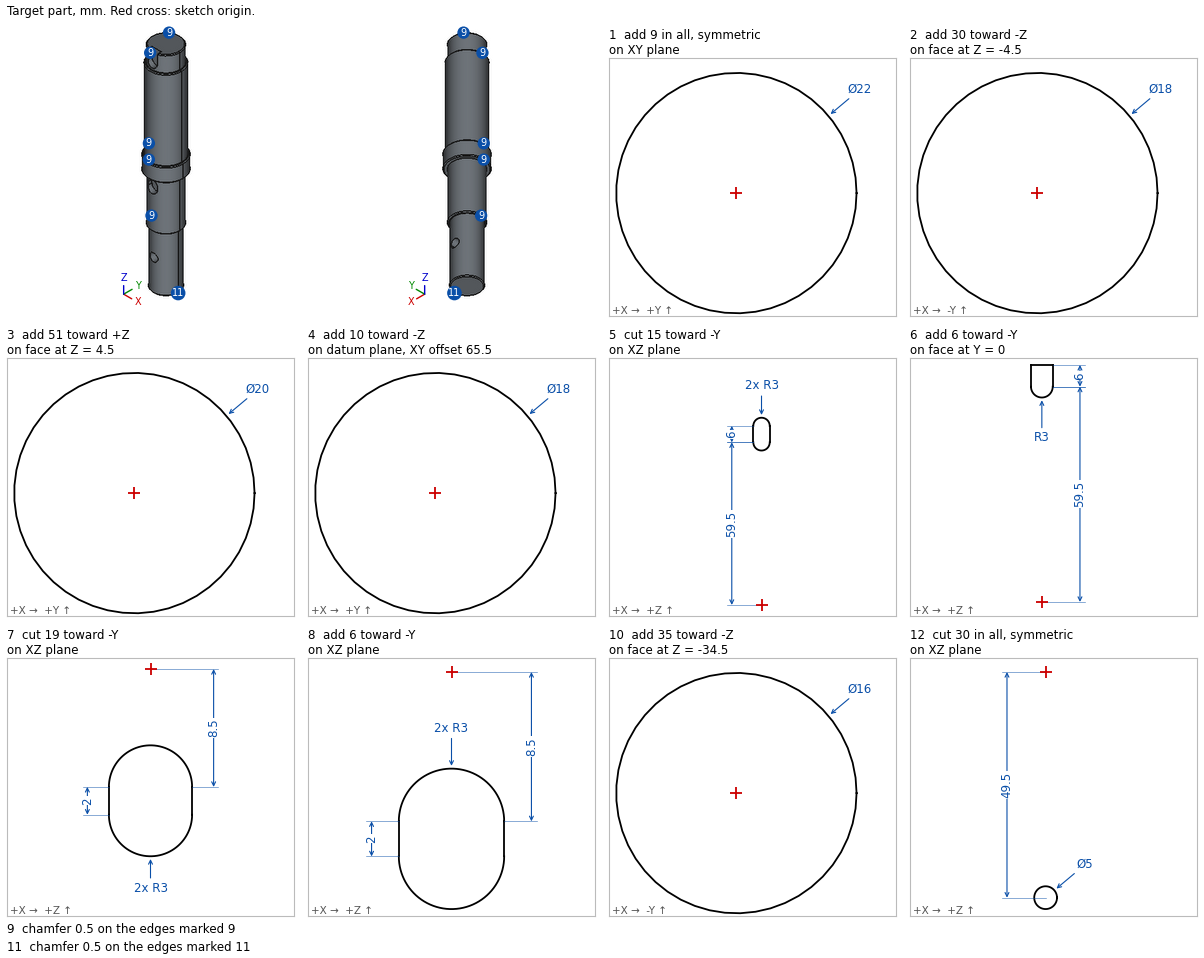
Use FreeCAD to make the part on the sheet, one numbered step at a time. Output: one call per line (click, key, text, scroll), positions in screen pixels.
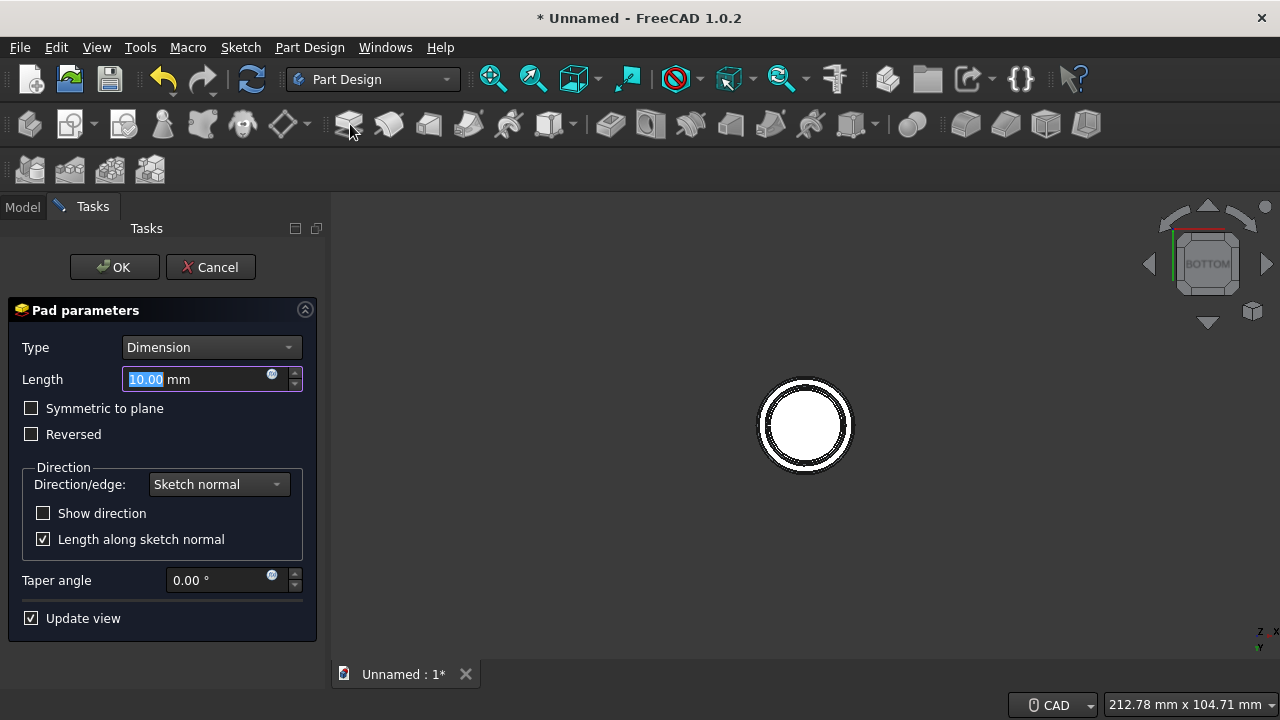
text(35)
key(Tab)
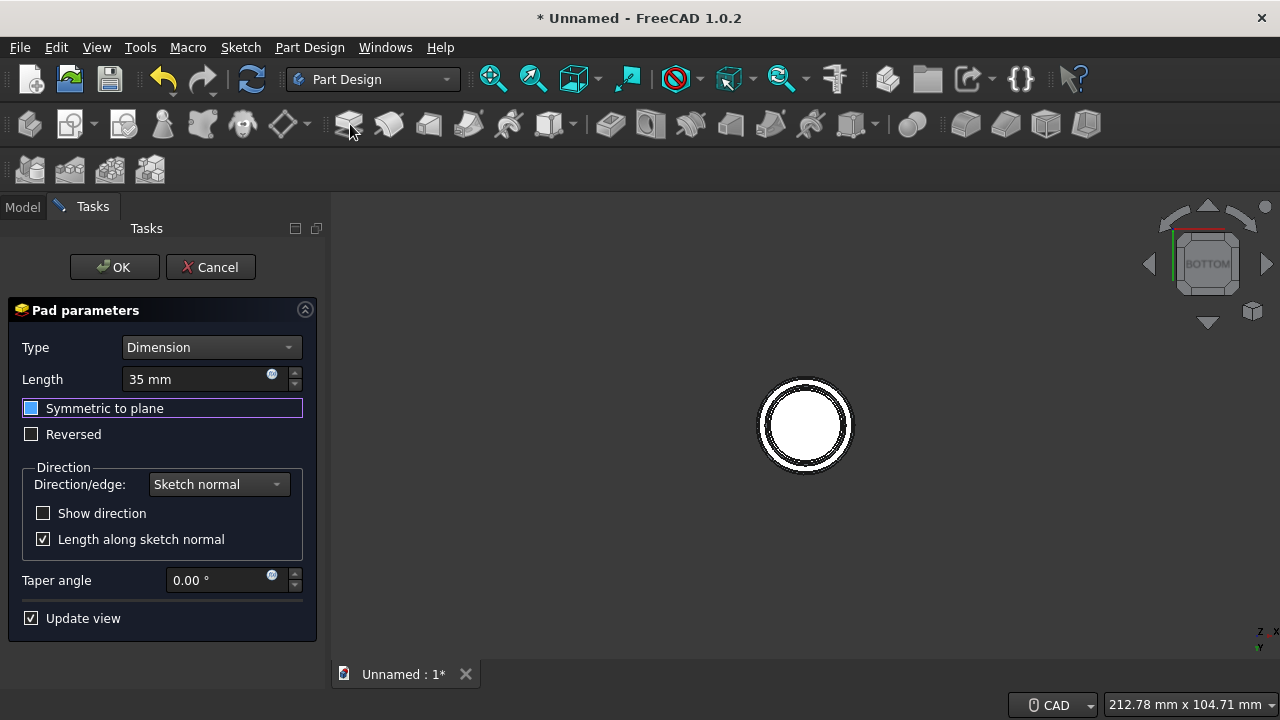
click(115, 267)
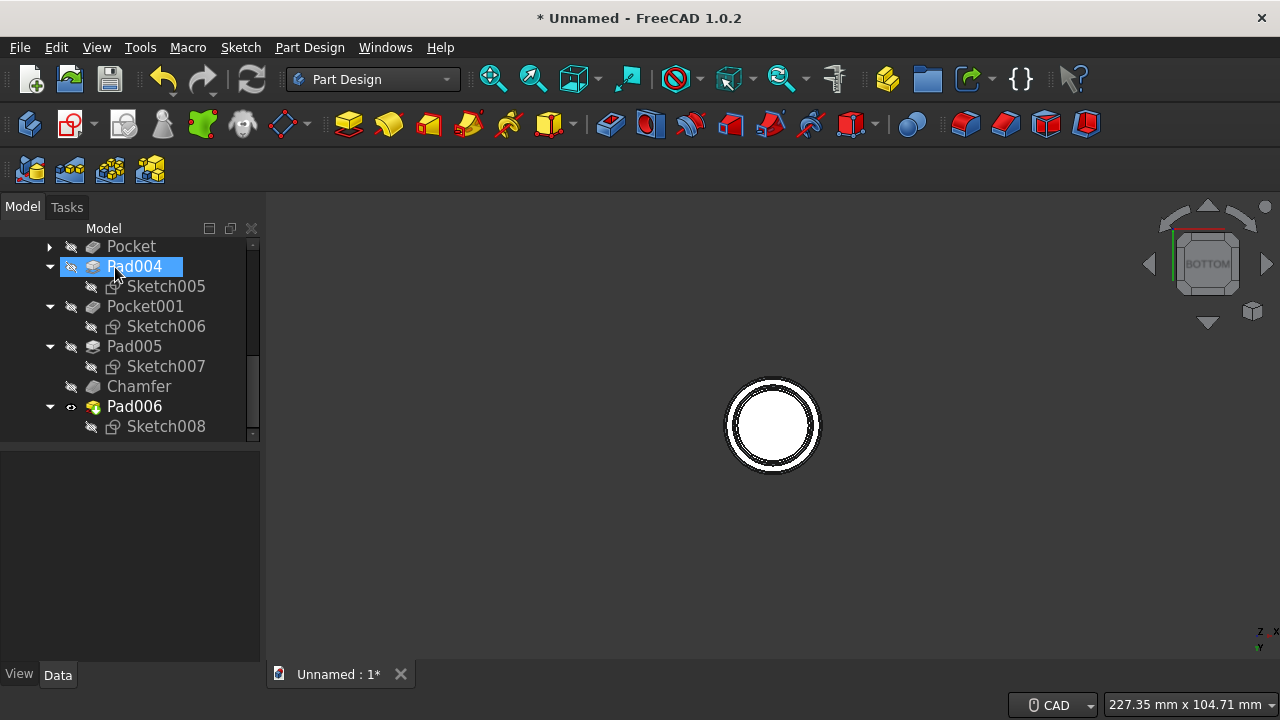
click(494, 80)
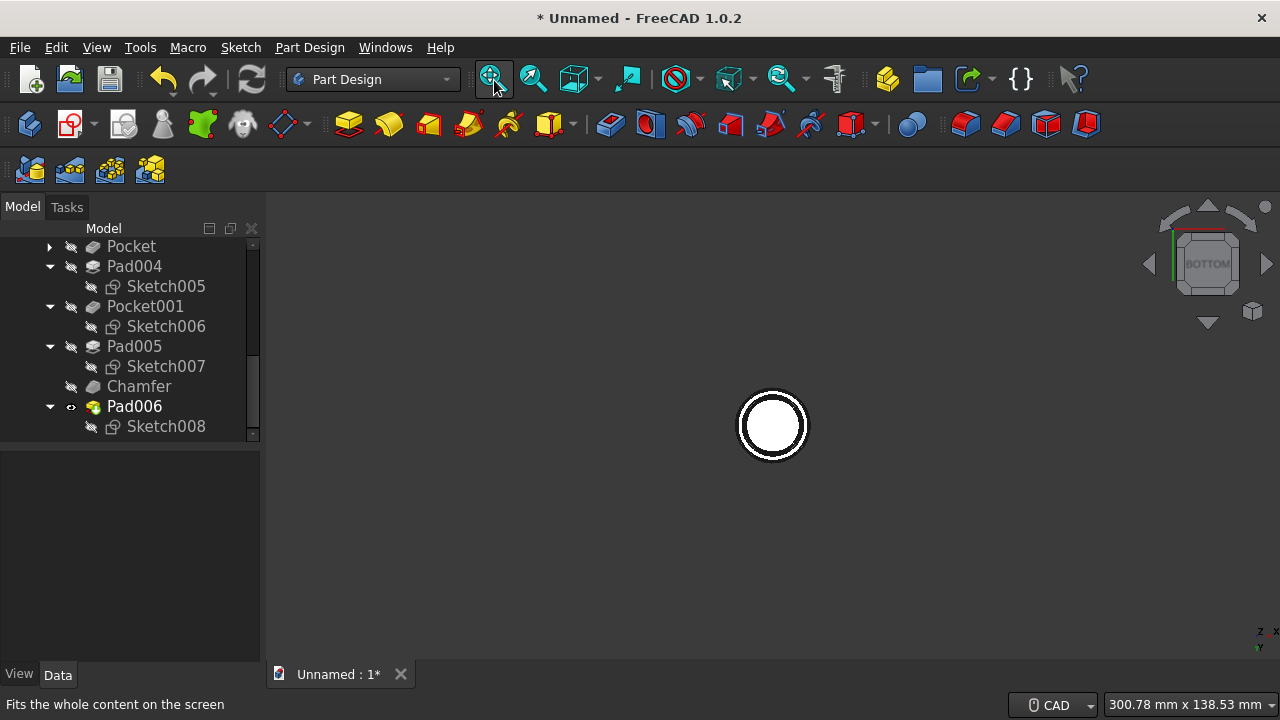
click(746, 424)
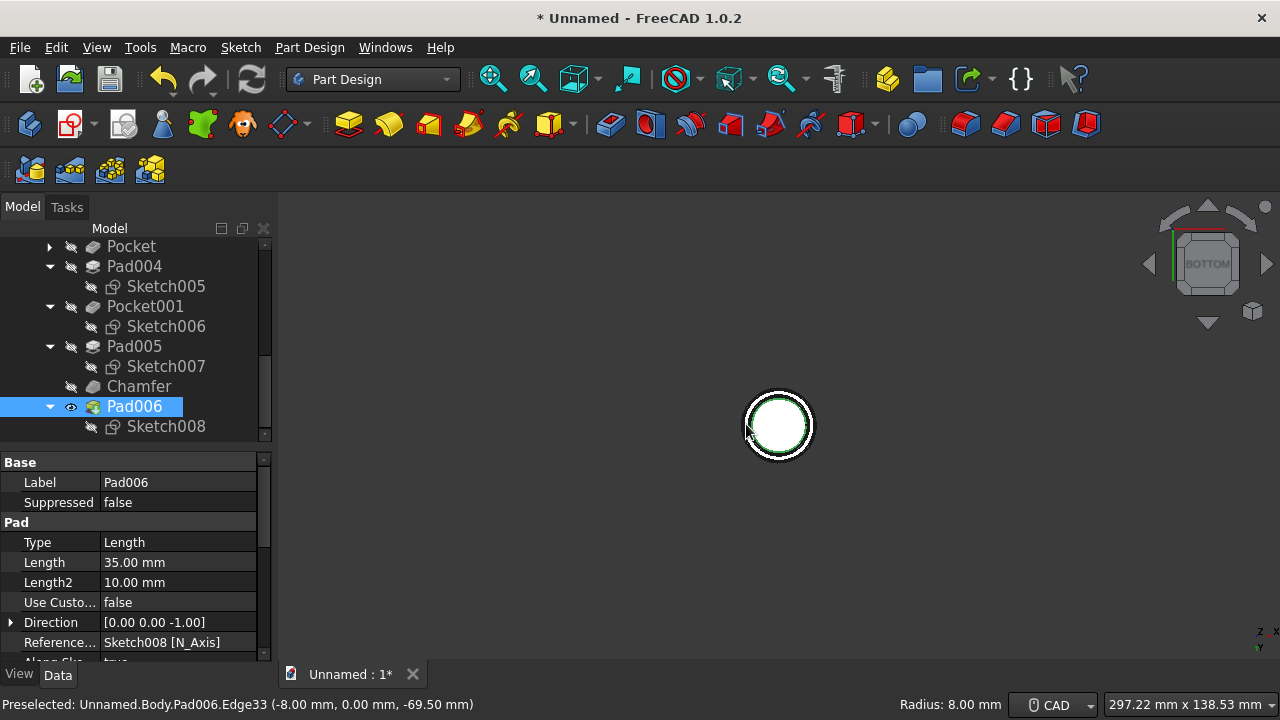
click(1006, 124)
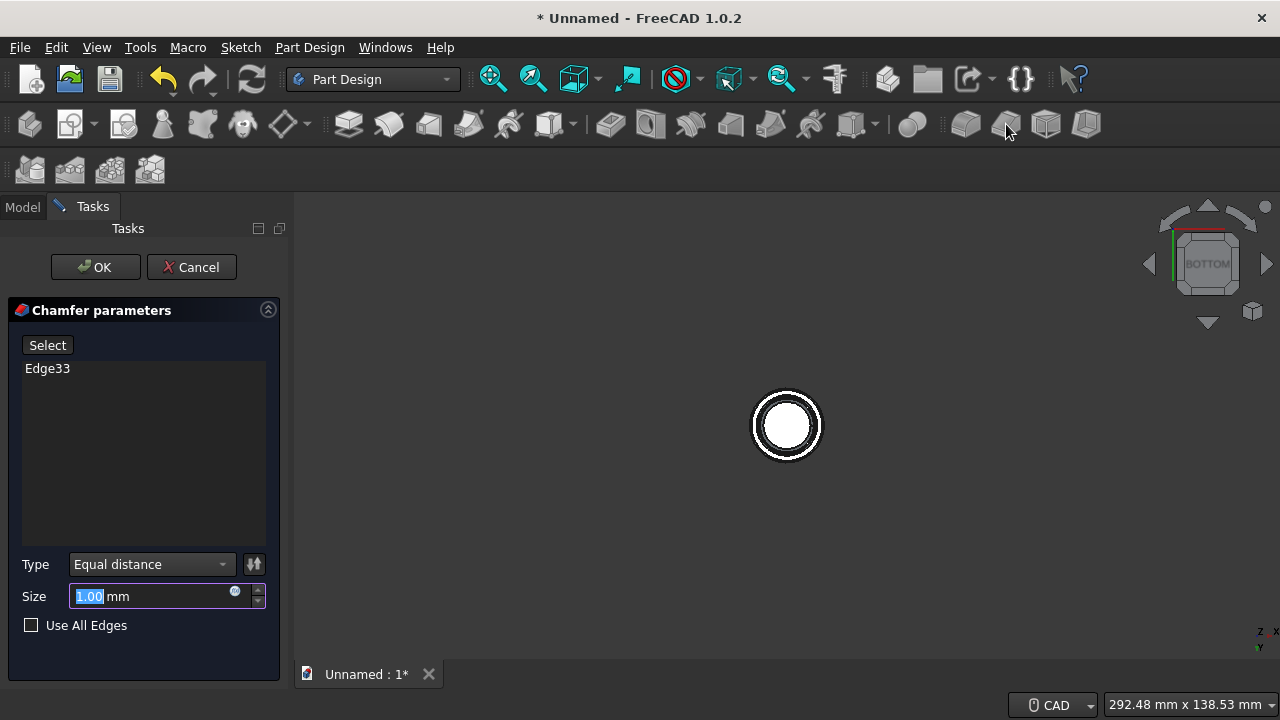
text(0.5)
key(Tab)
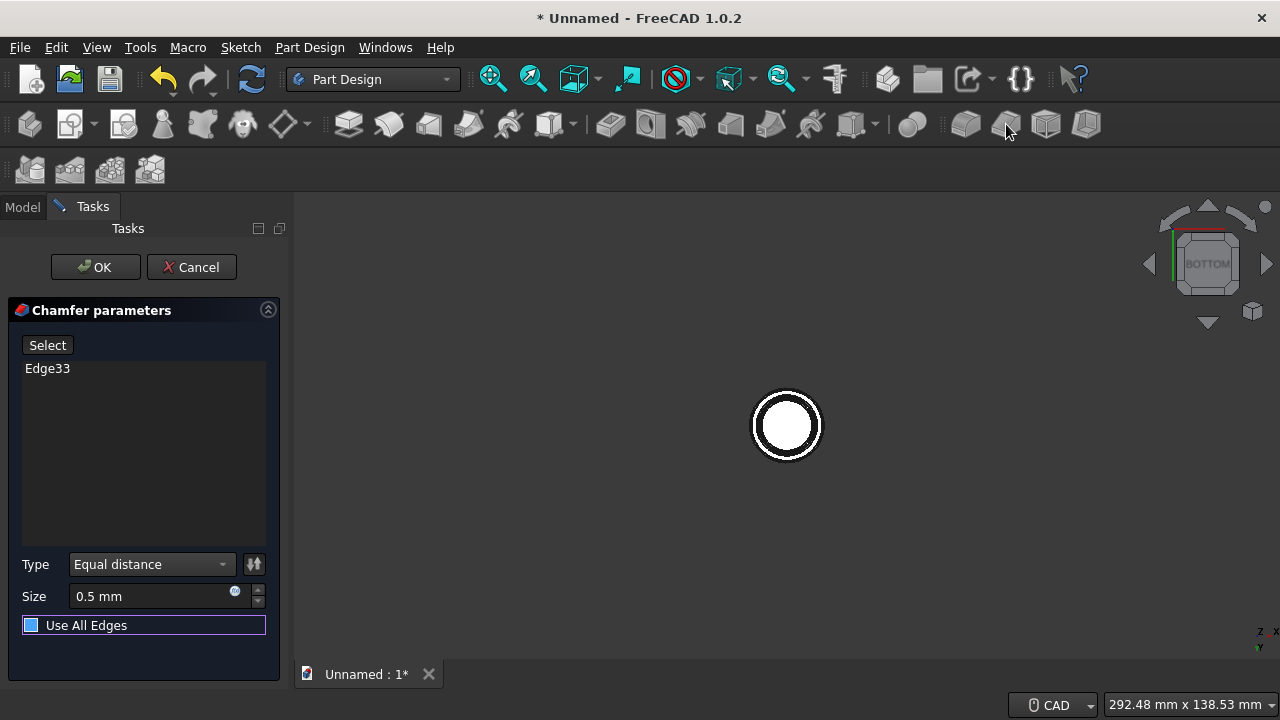
click(96, 267)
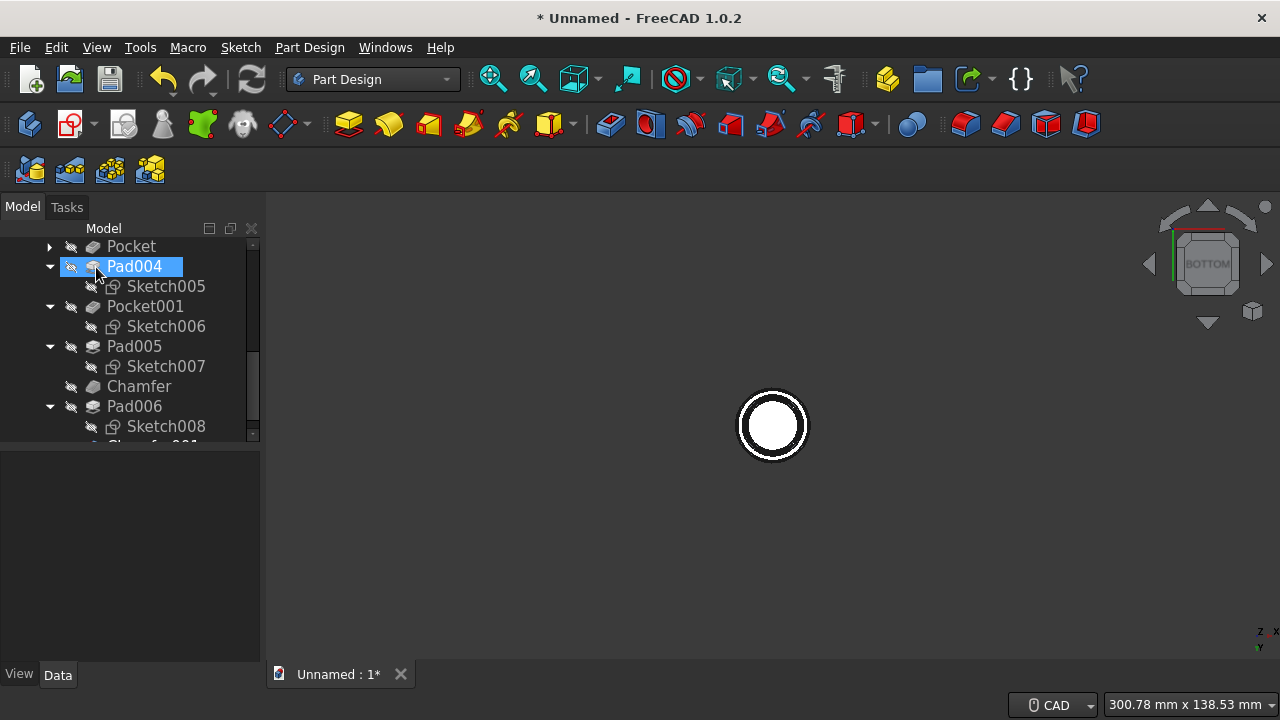
click(494, 80)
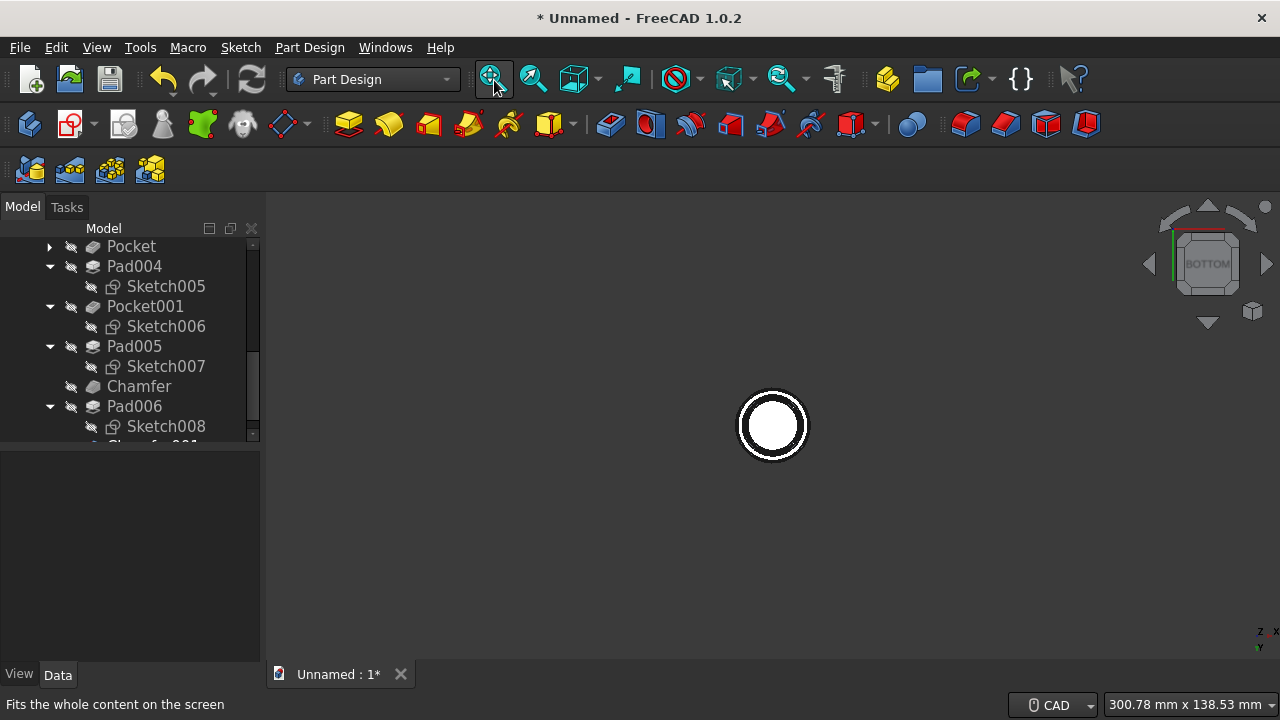
click(70, 124)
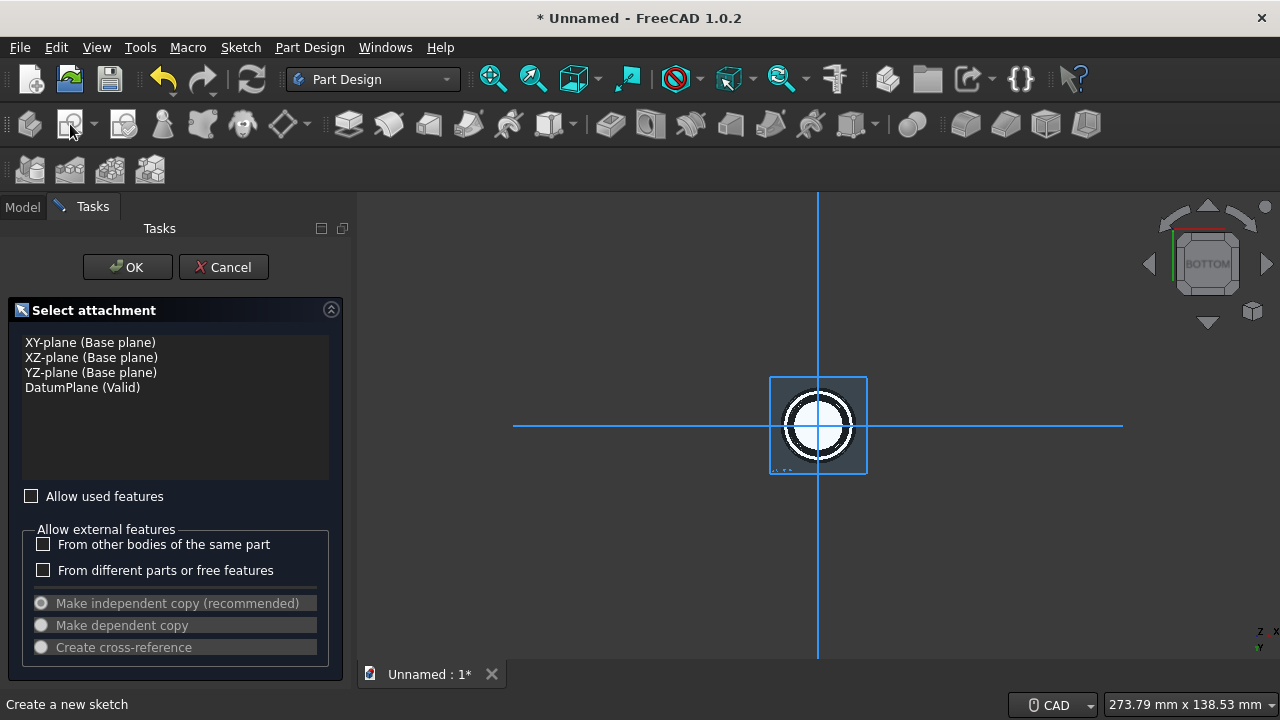
click(82, 358)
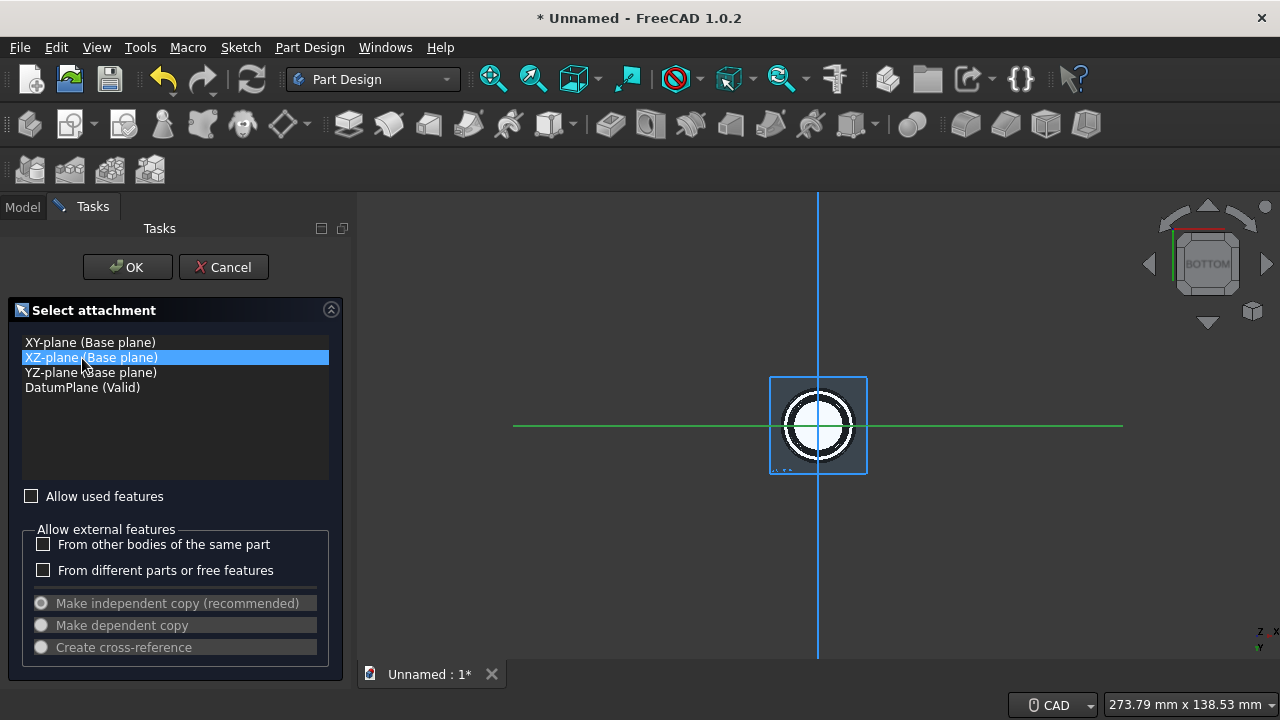
click(128, 267)